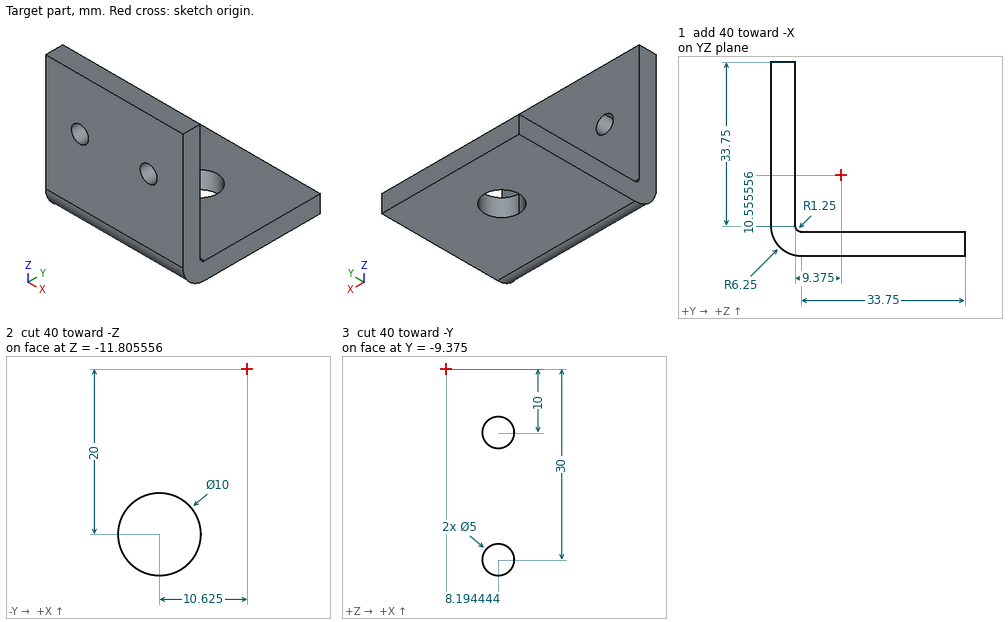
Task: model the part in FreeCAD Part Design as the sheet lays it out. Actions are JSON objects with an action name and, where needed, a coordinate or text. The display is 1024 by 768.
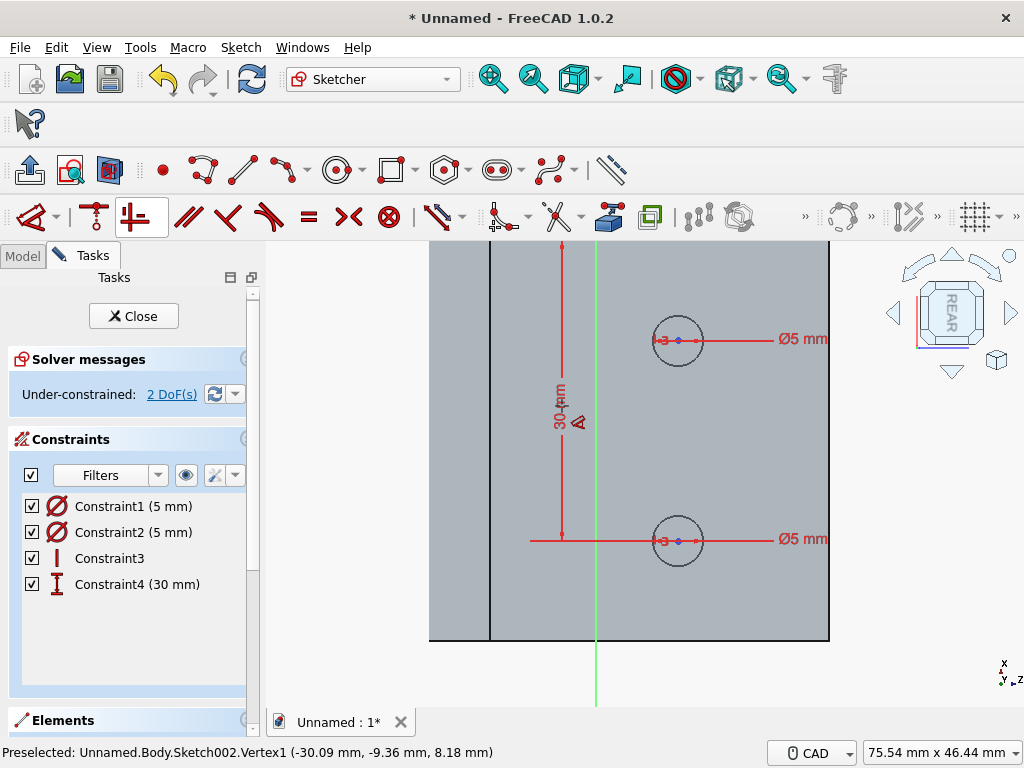
{"action": "left_click", "coordinate": [678, 341]}
{"action": "left_click", "coordinate": [562, 305]}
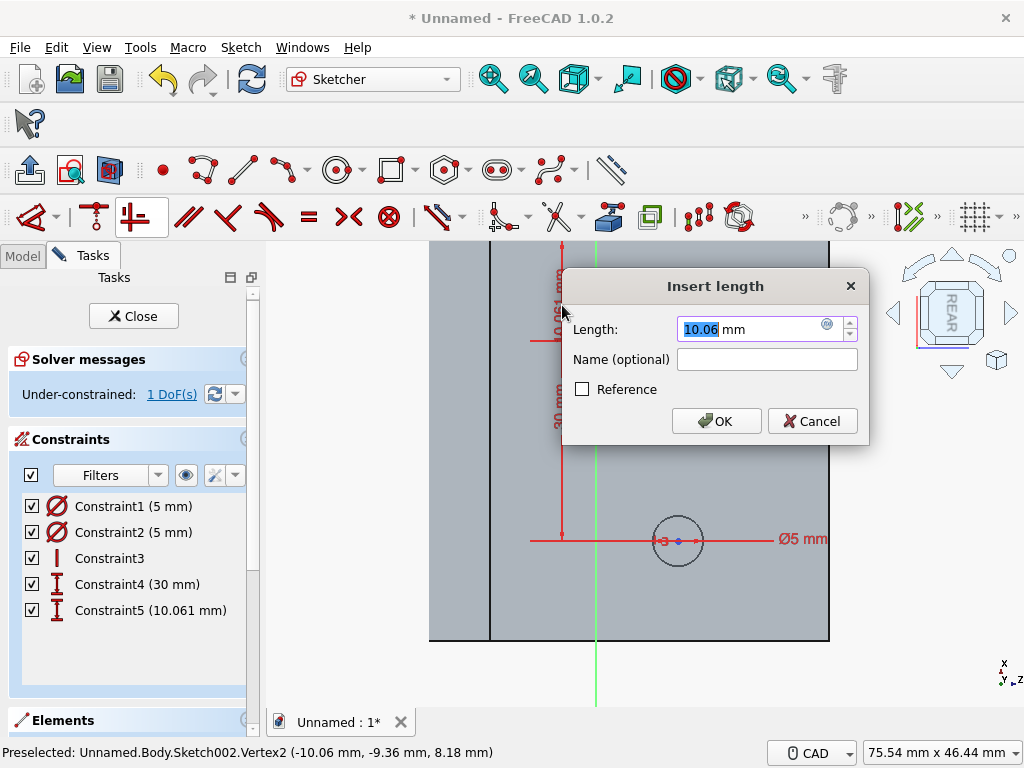
{"action": "type", "text": "10"}
{"action": "key", "text": "Return"}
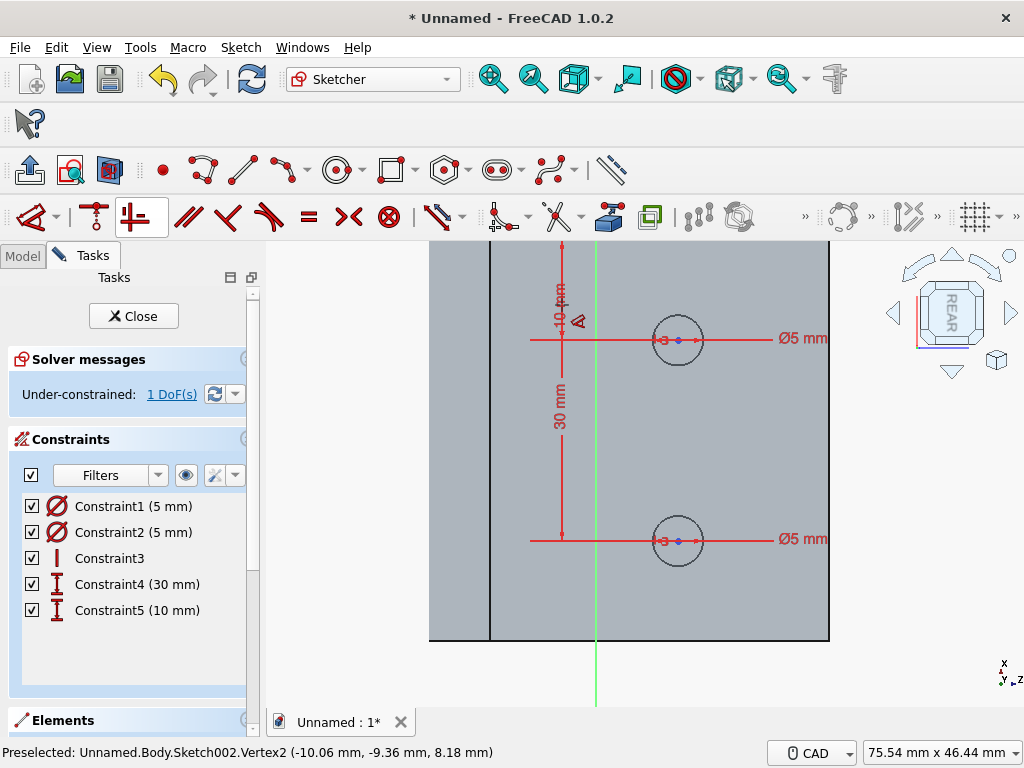
{"action": "left_click", "coordinate": [678, 541]}
{"action": "left_click", "coordinate": [637, 575]}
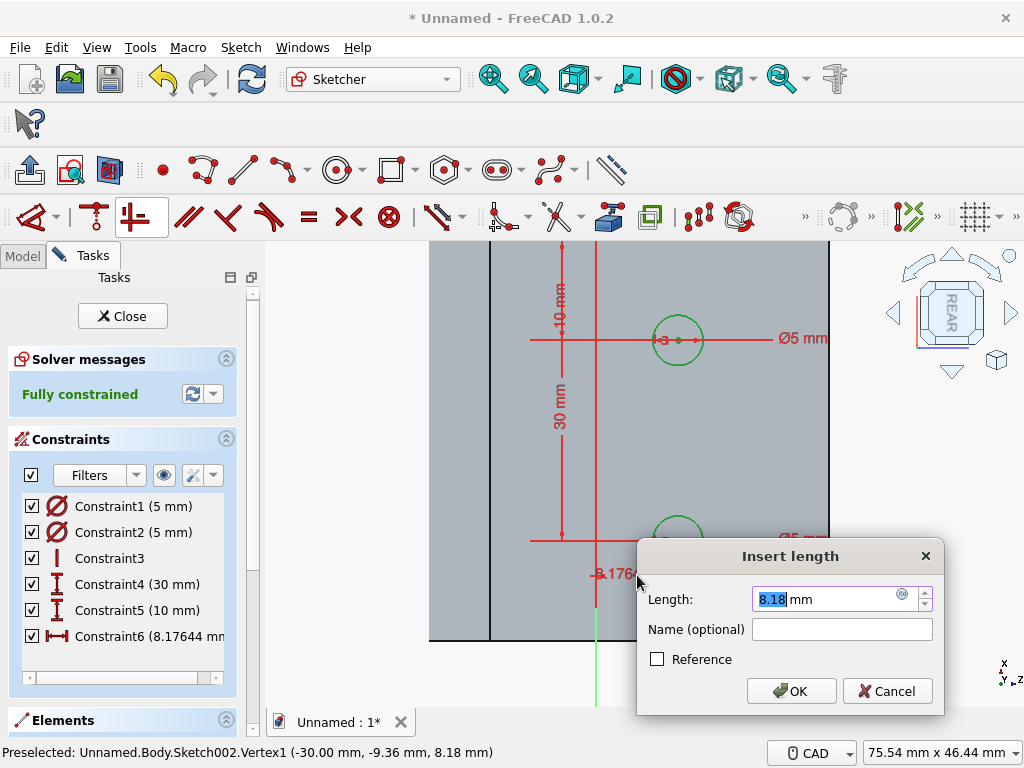
{"action": "type", "text": "8.194444"}
{"action": "key", "text": "Return"}
{"action": "key", "text": "Escape"}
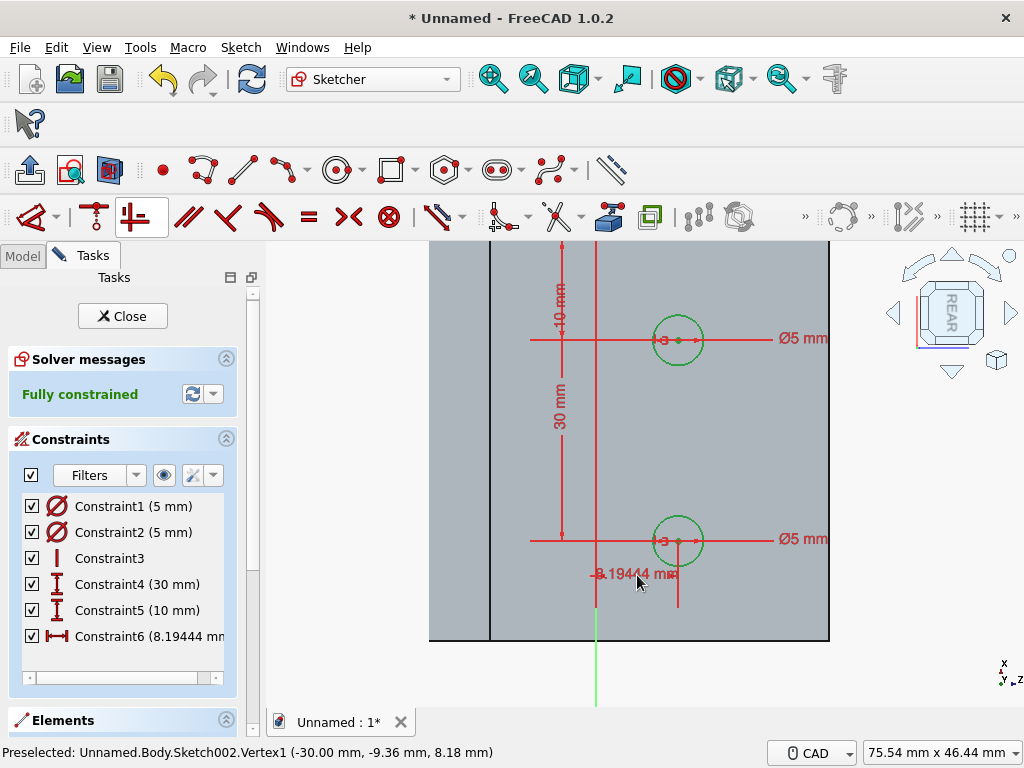
{"action": "left_click", "coordinate": [123, 316]}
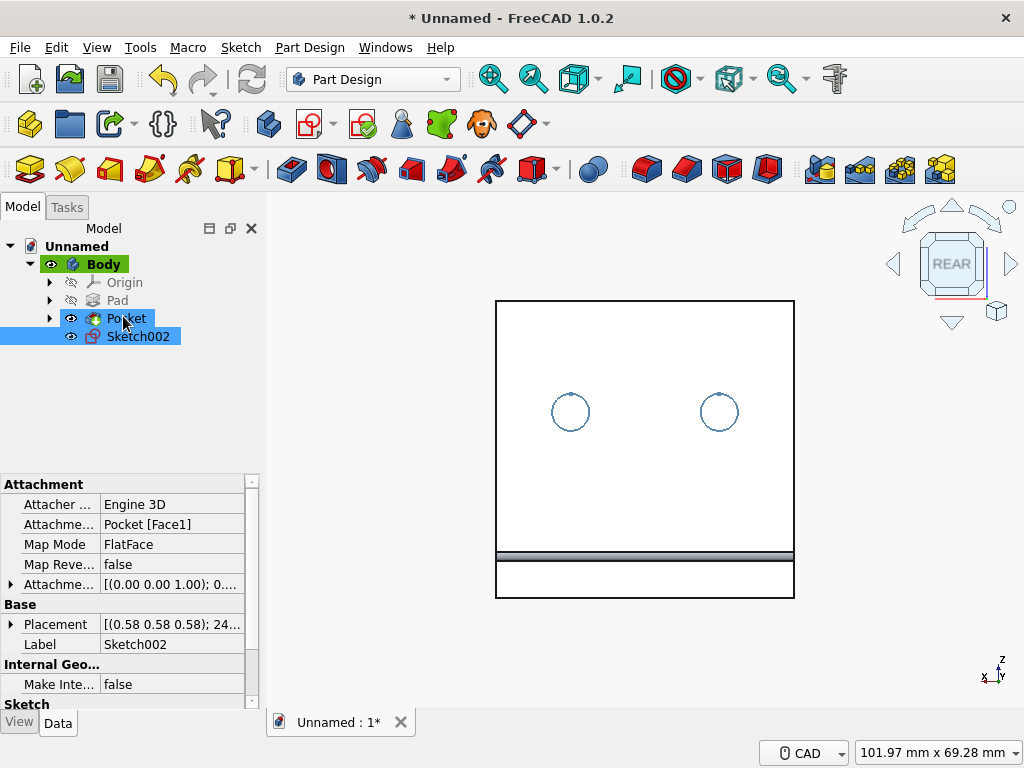
{"action": "left_click", "coordinate": [292, 170]}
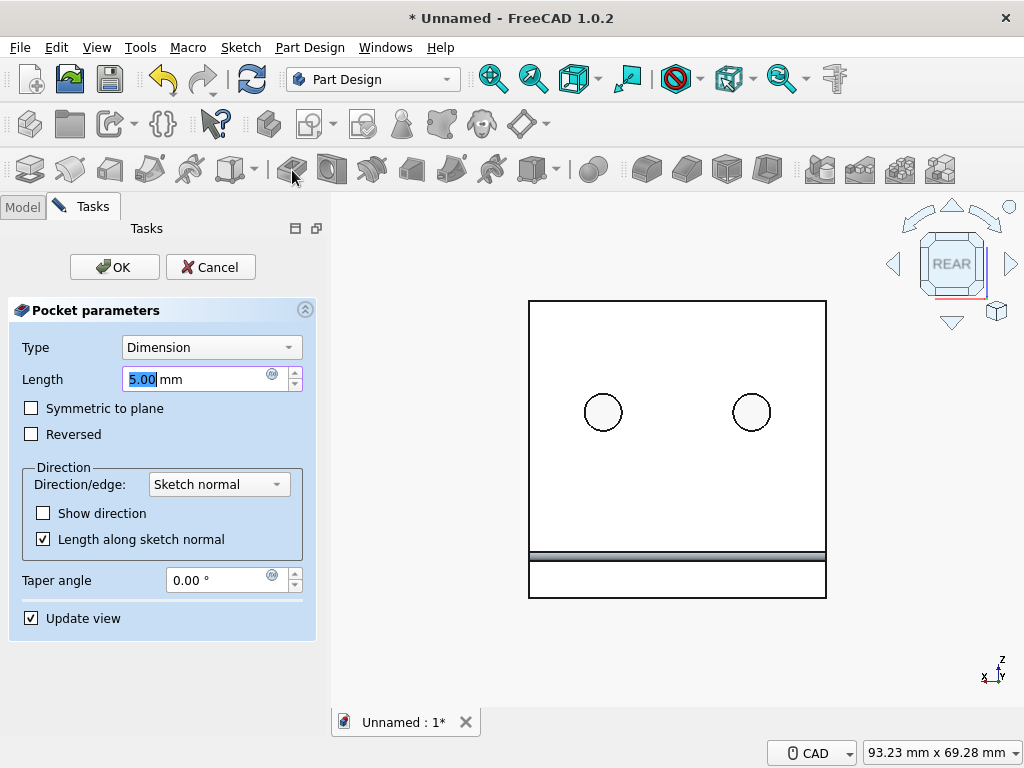
{"action": "type", "text": "40"}
{"action": "key", "text": "Tab"}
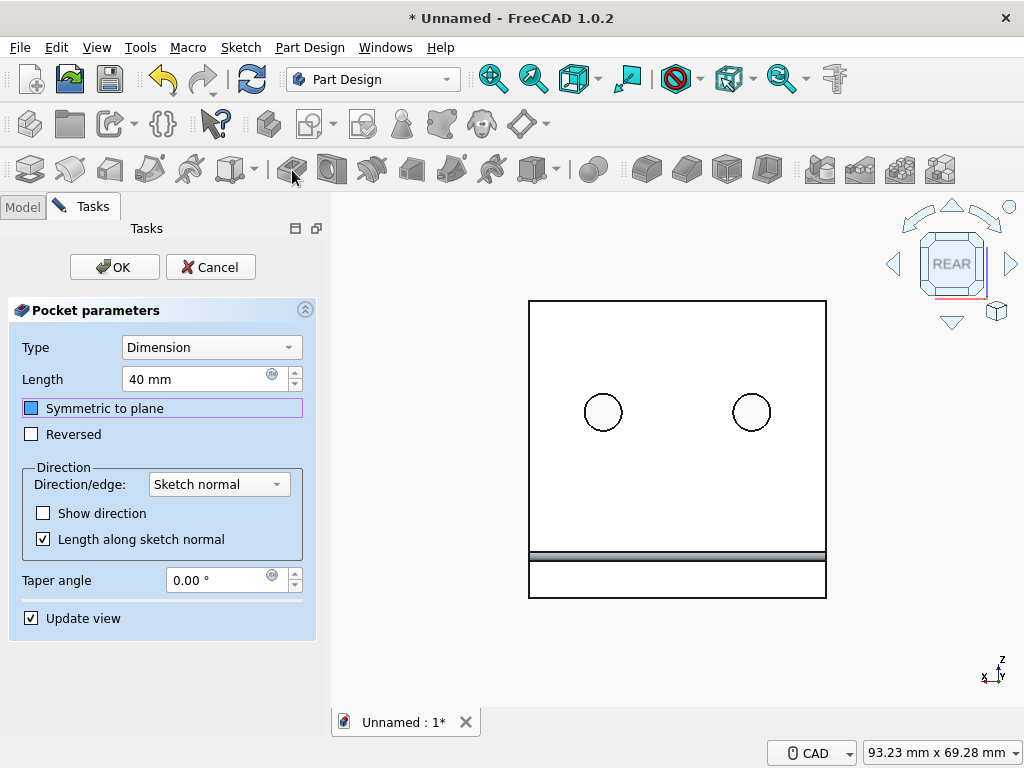
{"action": "left_click", "coordinate": [115, 267]}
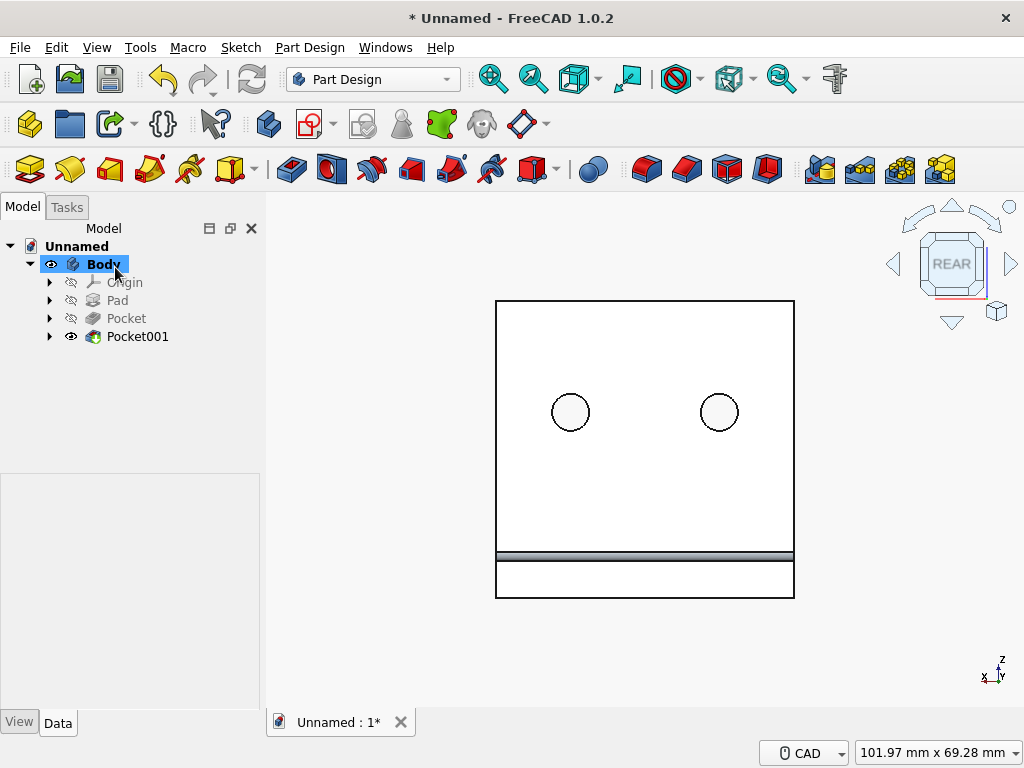
{"action": "key", "text": "0"}